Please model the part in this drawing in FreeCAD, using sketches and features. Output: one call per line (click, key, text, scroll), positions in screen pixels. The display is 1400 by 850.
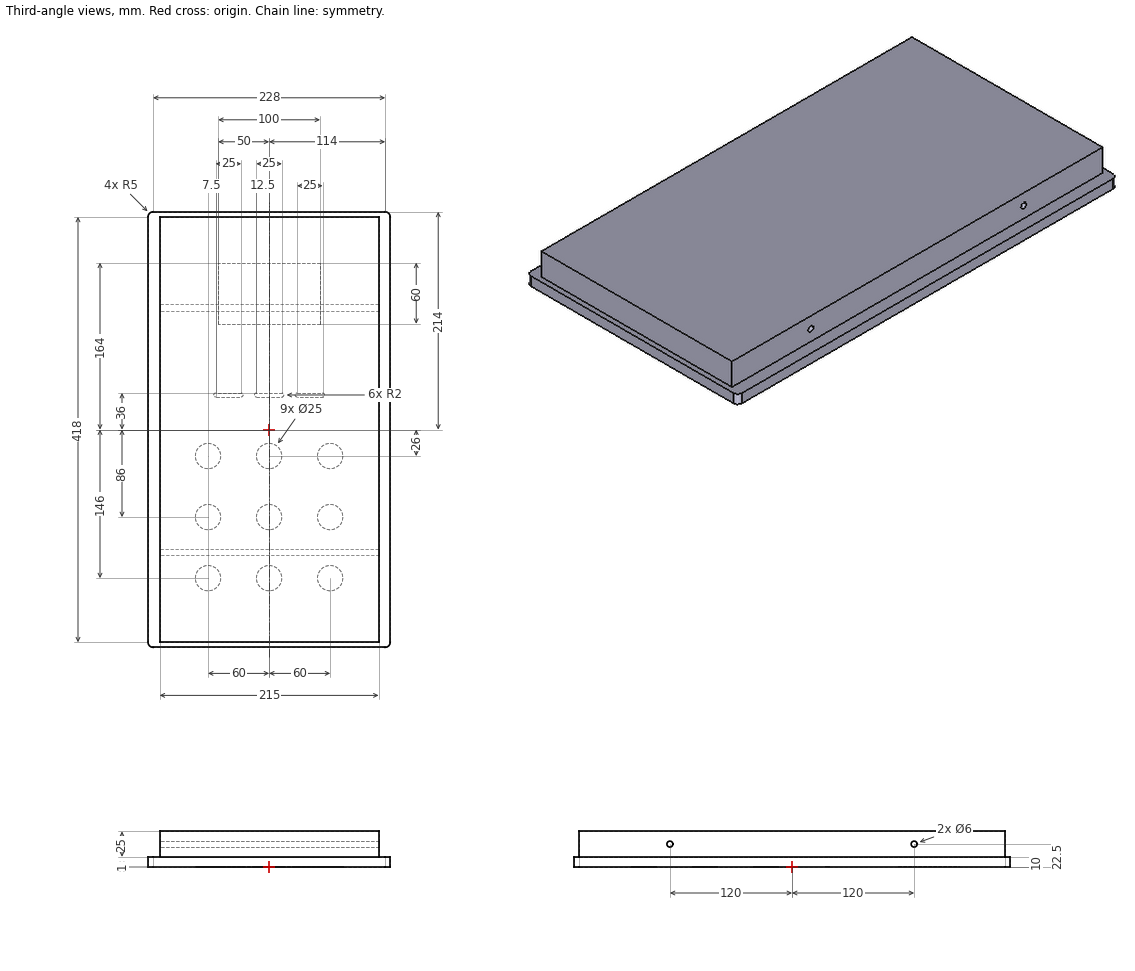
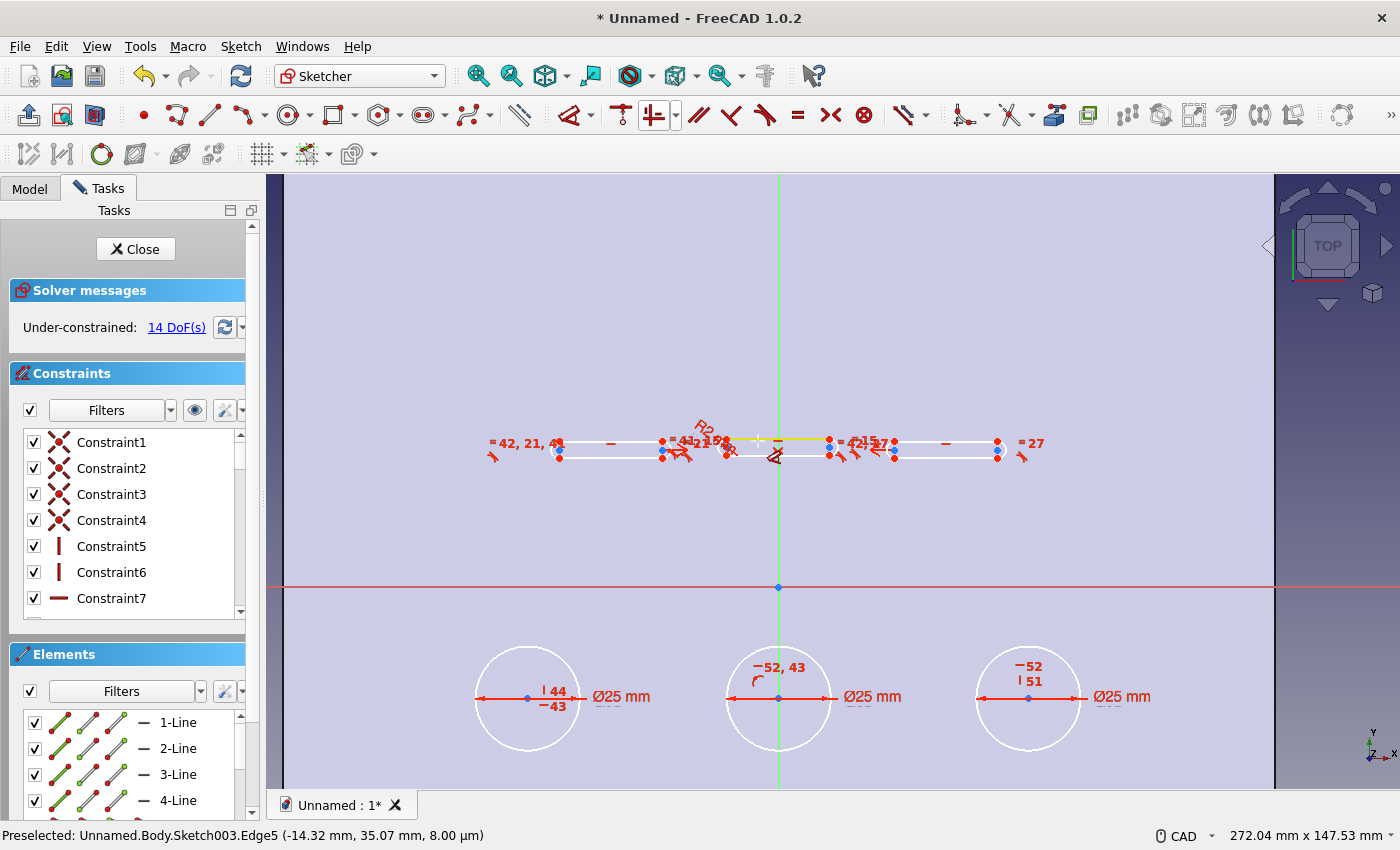
click(757, 439)
click(754, 405)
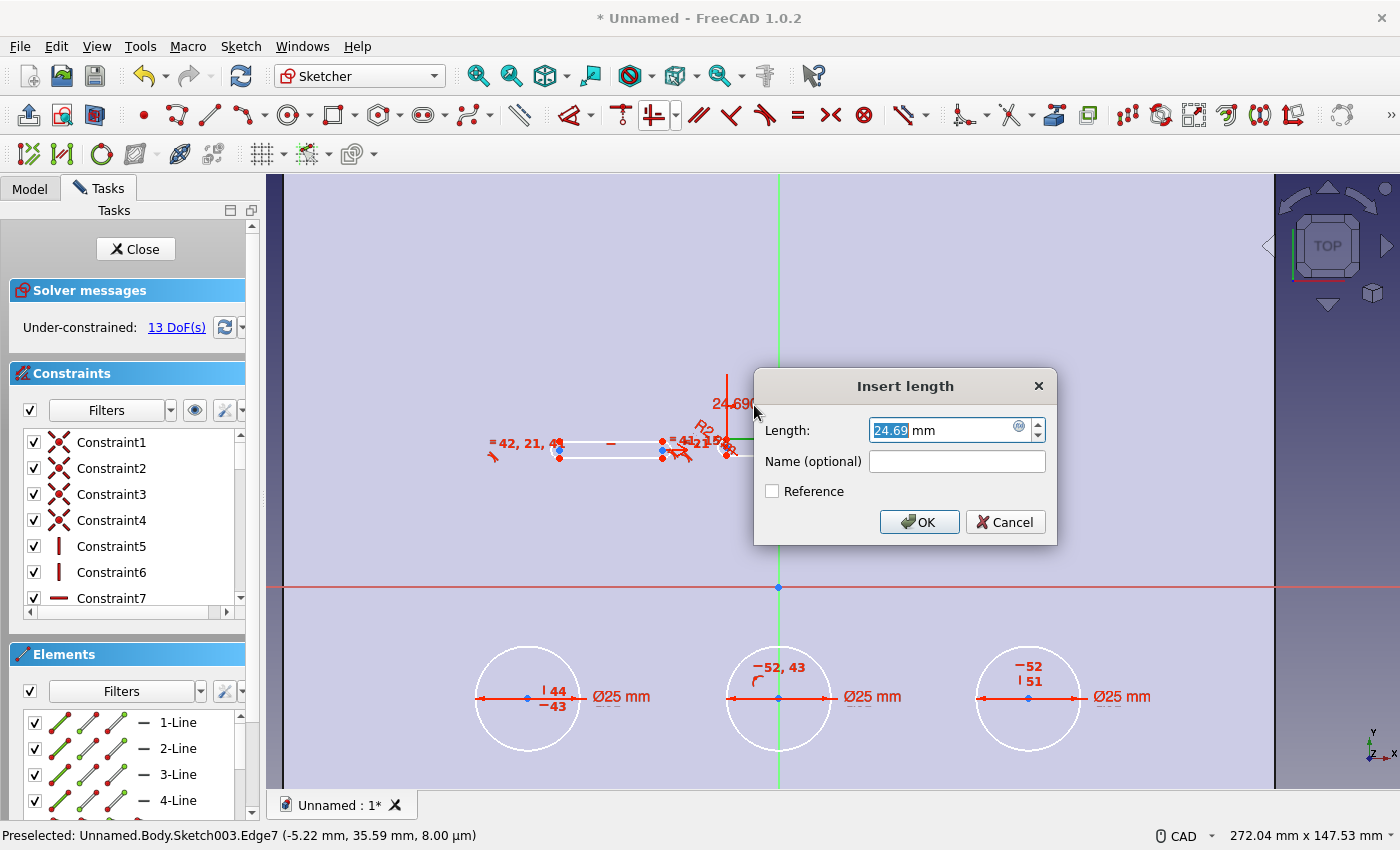
text(25)
key(Return)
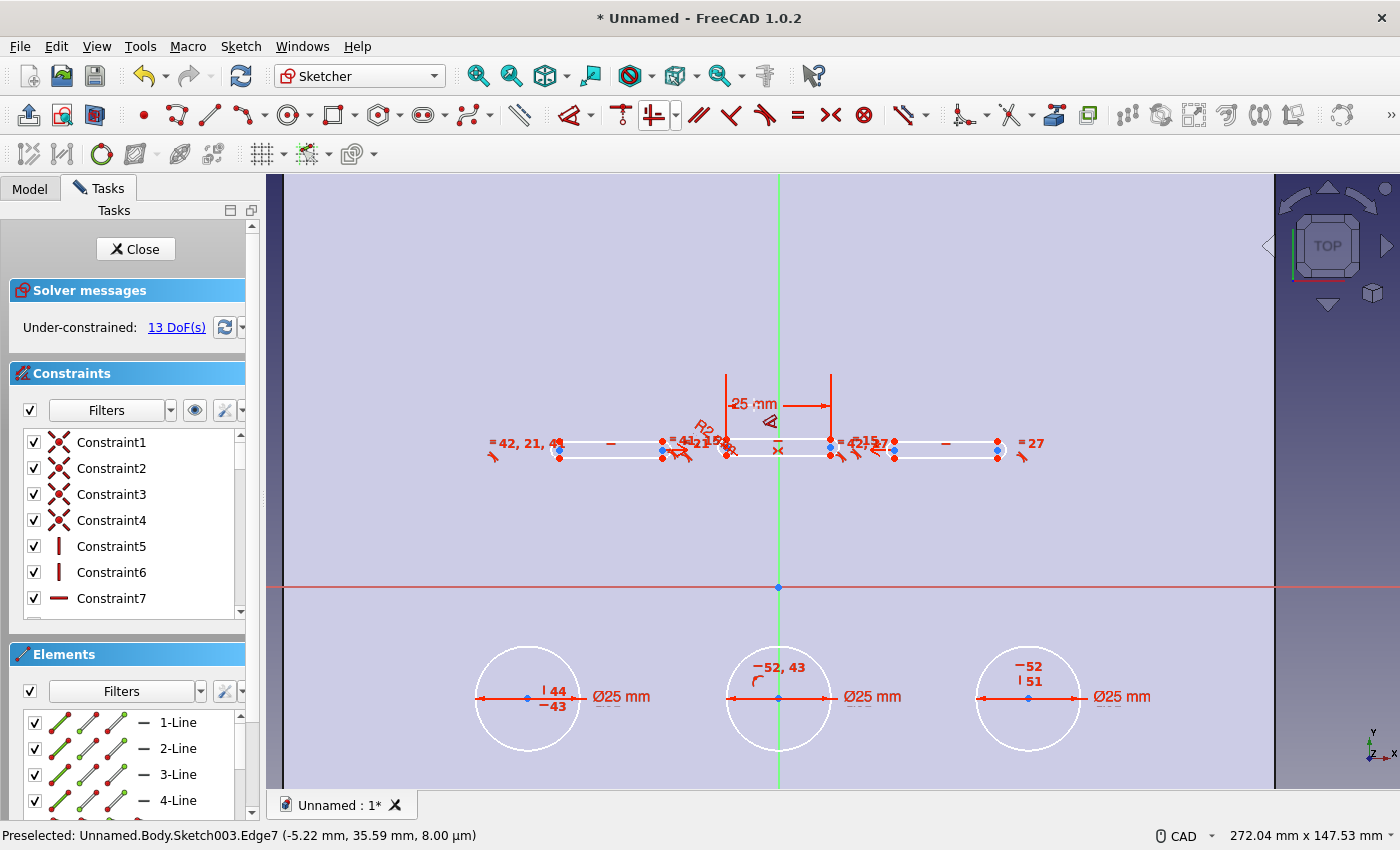
click(590, 442)
click(611, 408)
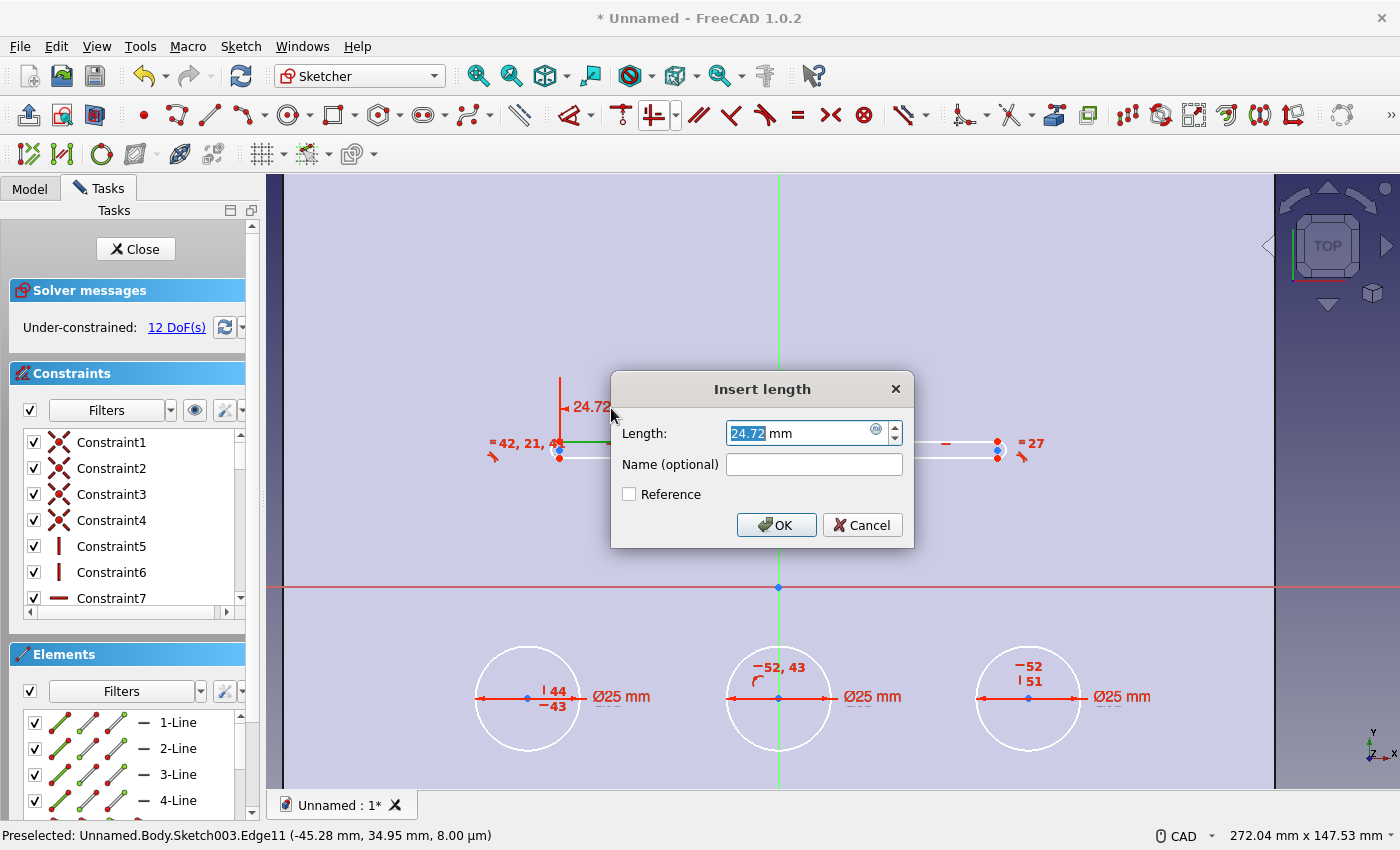
text(25)
key(Return)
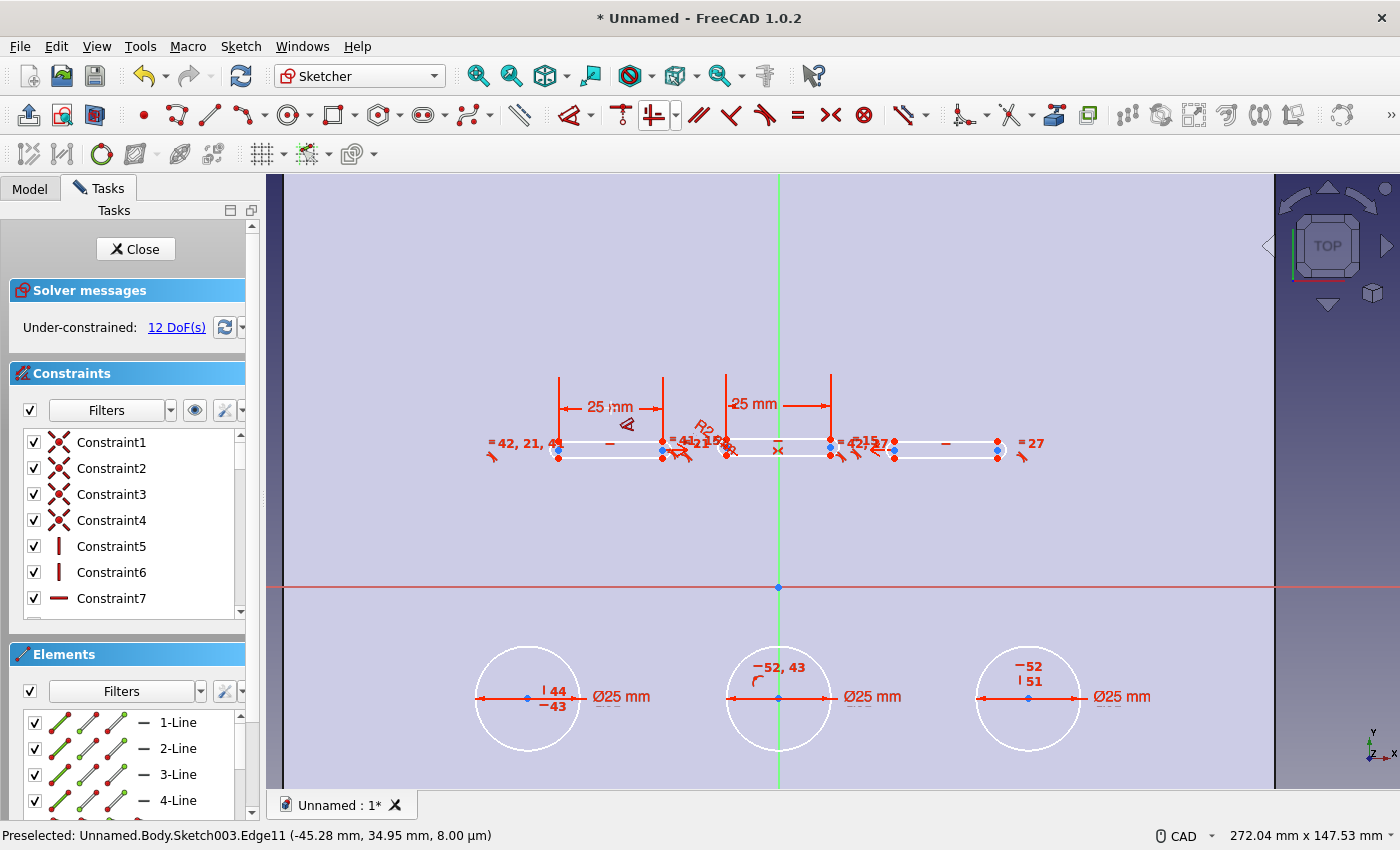
click(926, 442)
click(946, 408)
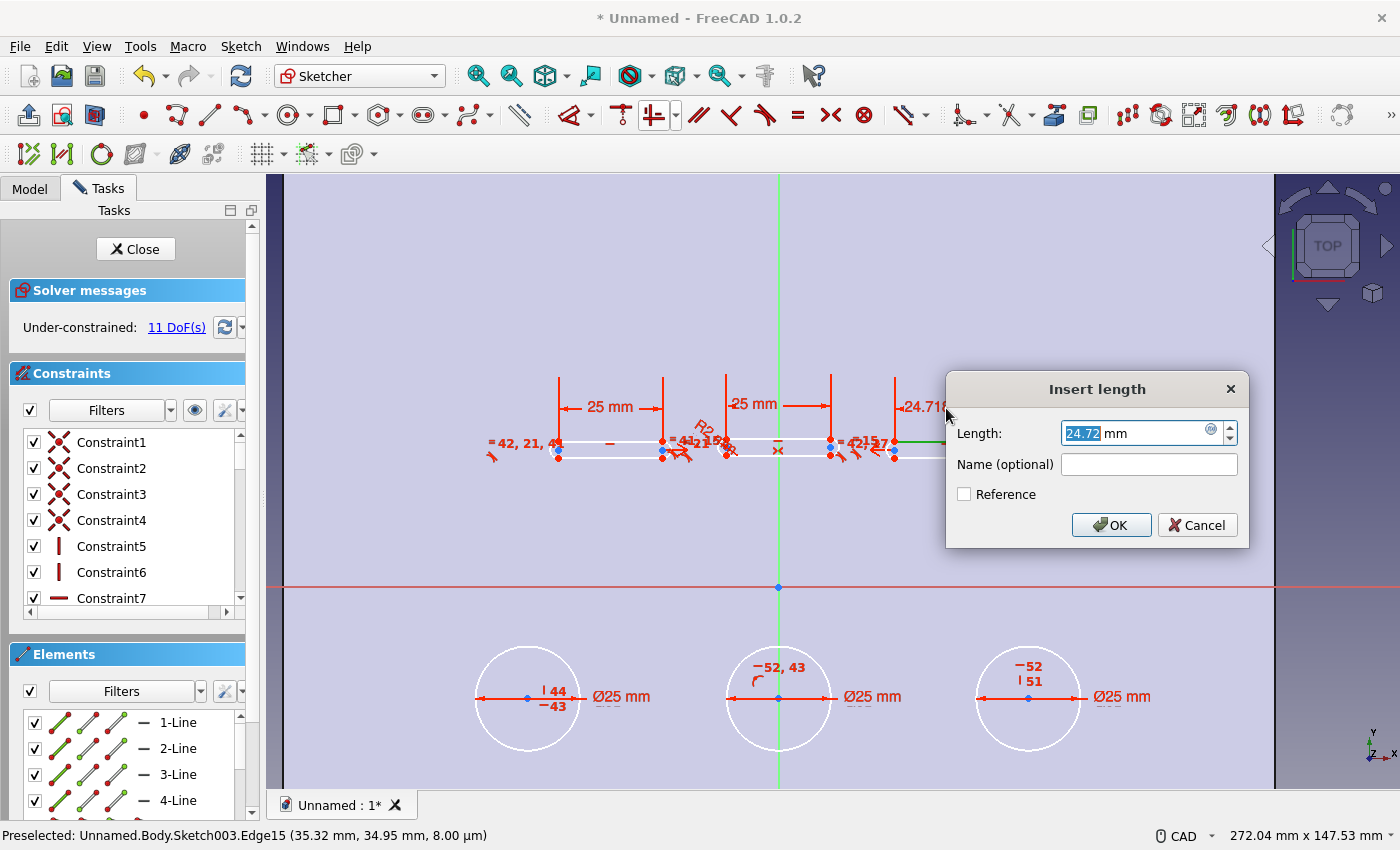
text(25)
key(Return)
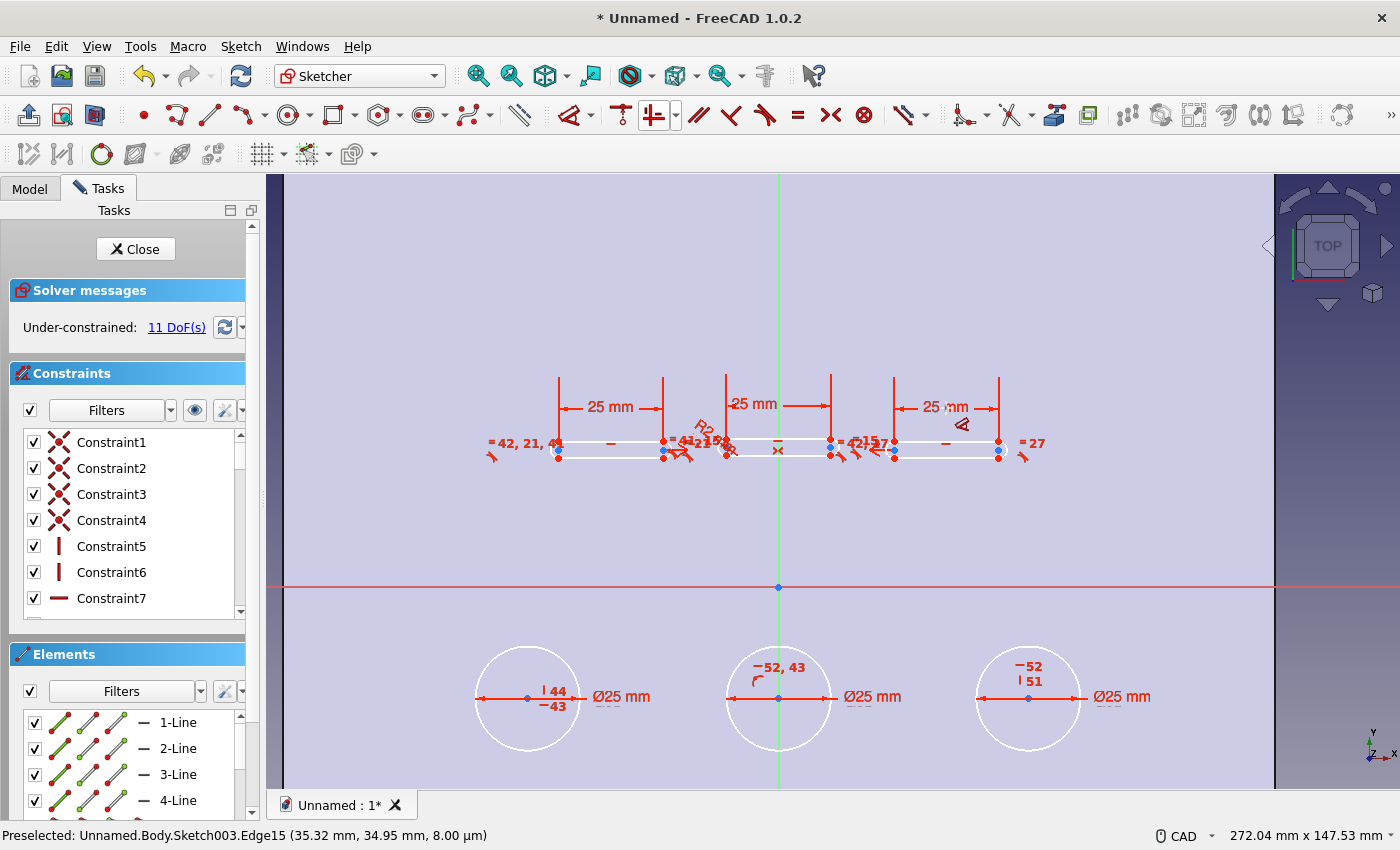
click(779, 699)
click(813, 643)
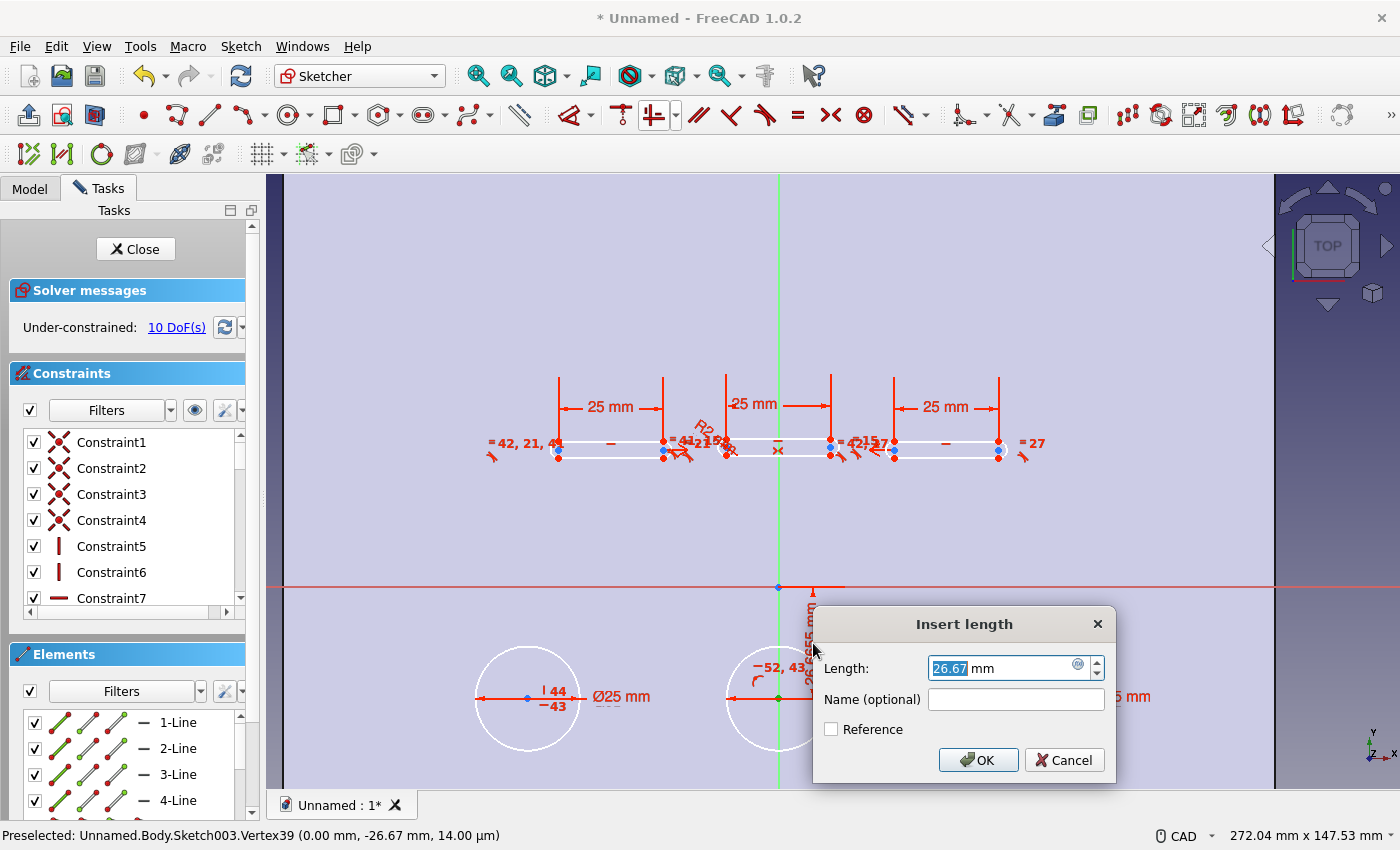
text(26)
key(Return)